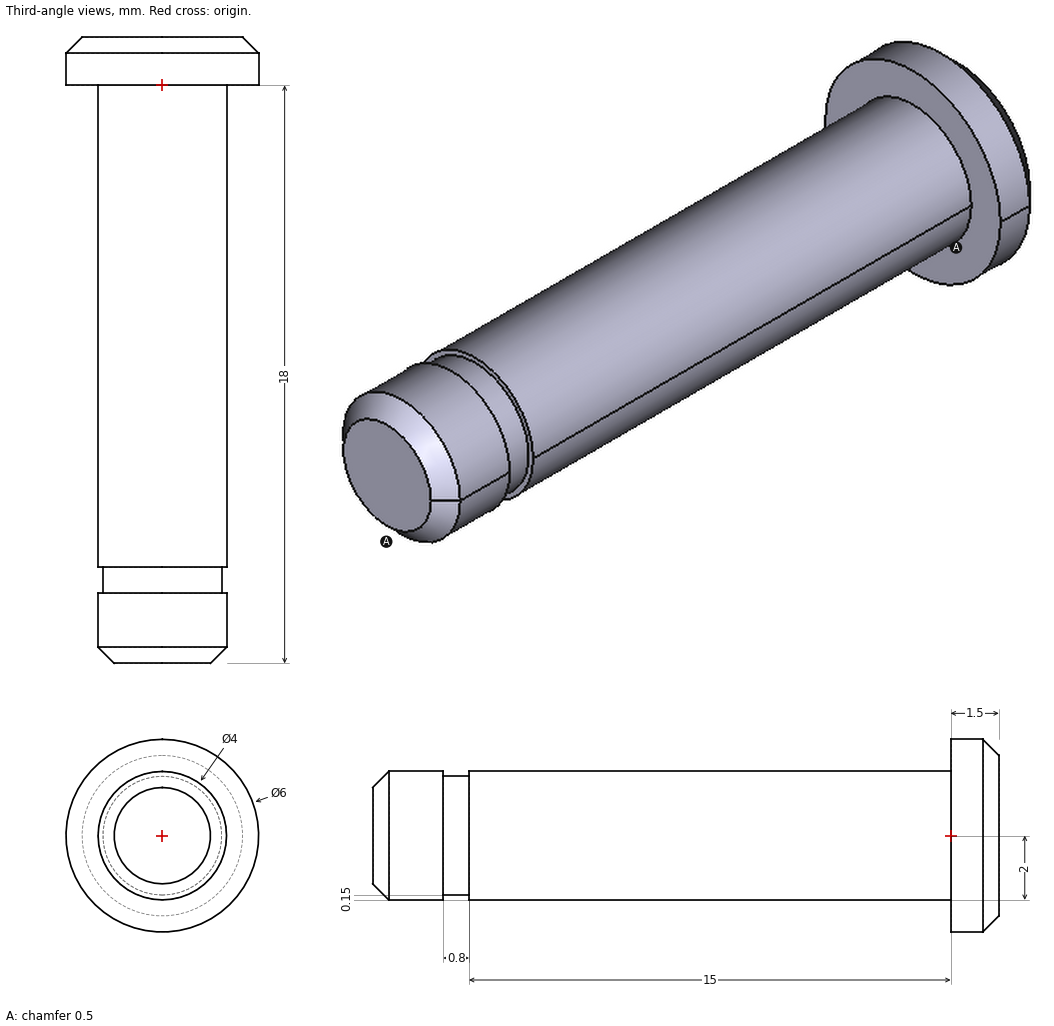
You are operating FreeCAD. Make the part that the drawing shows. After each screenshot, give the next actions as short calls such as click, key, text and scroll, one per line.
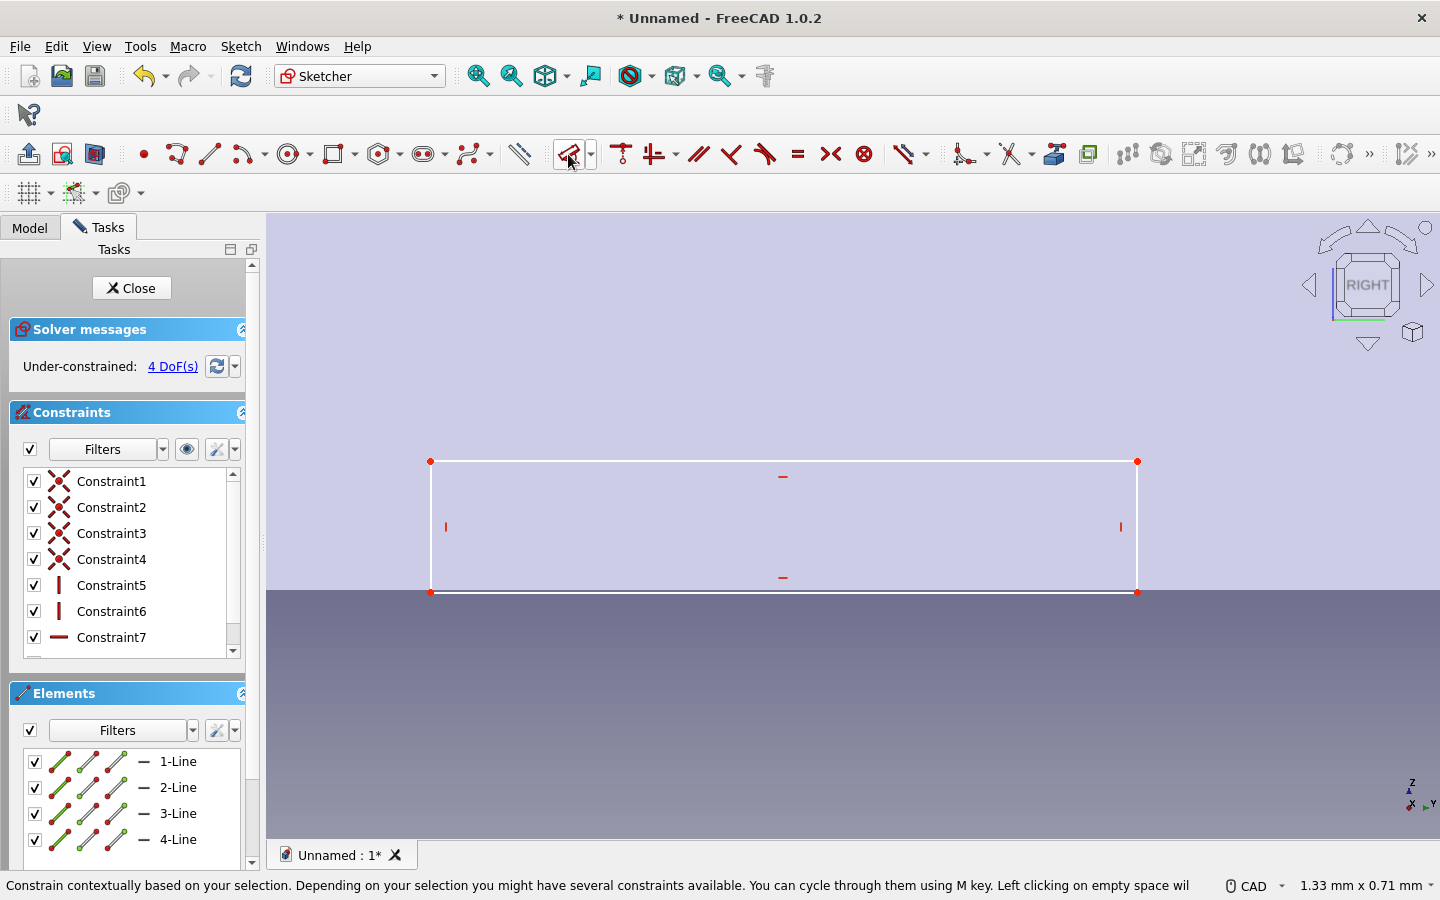
click(431, 593)
click(397, 417)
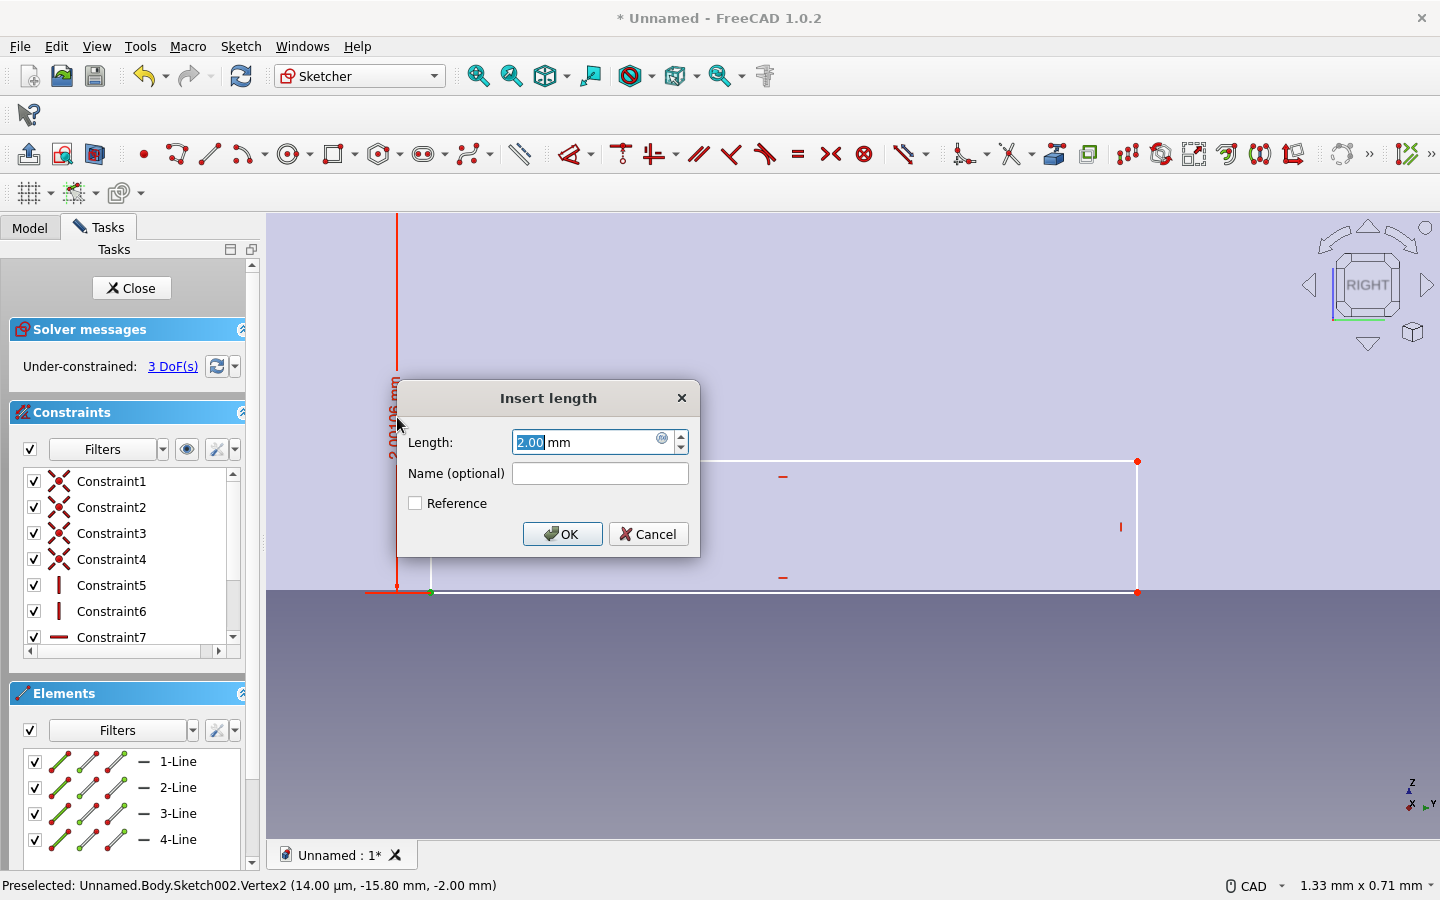
text(2)
key(Return)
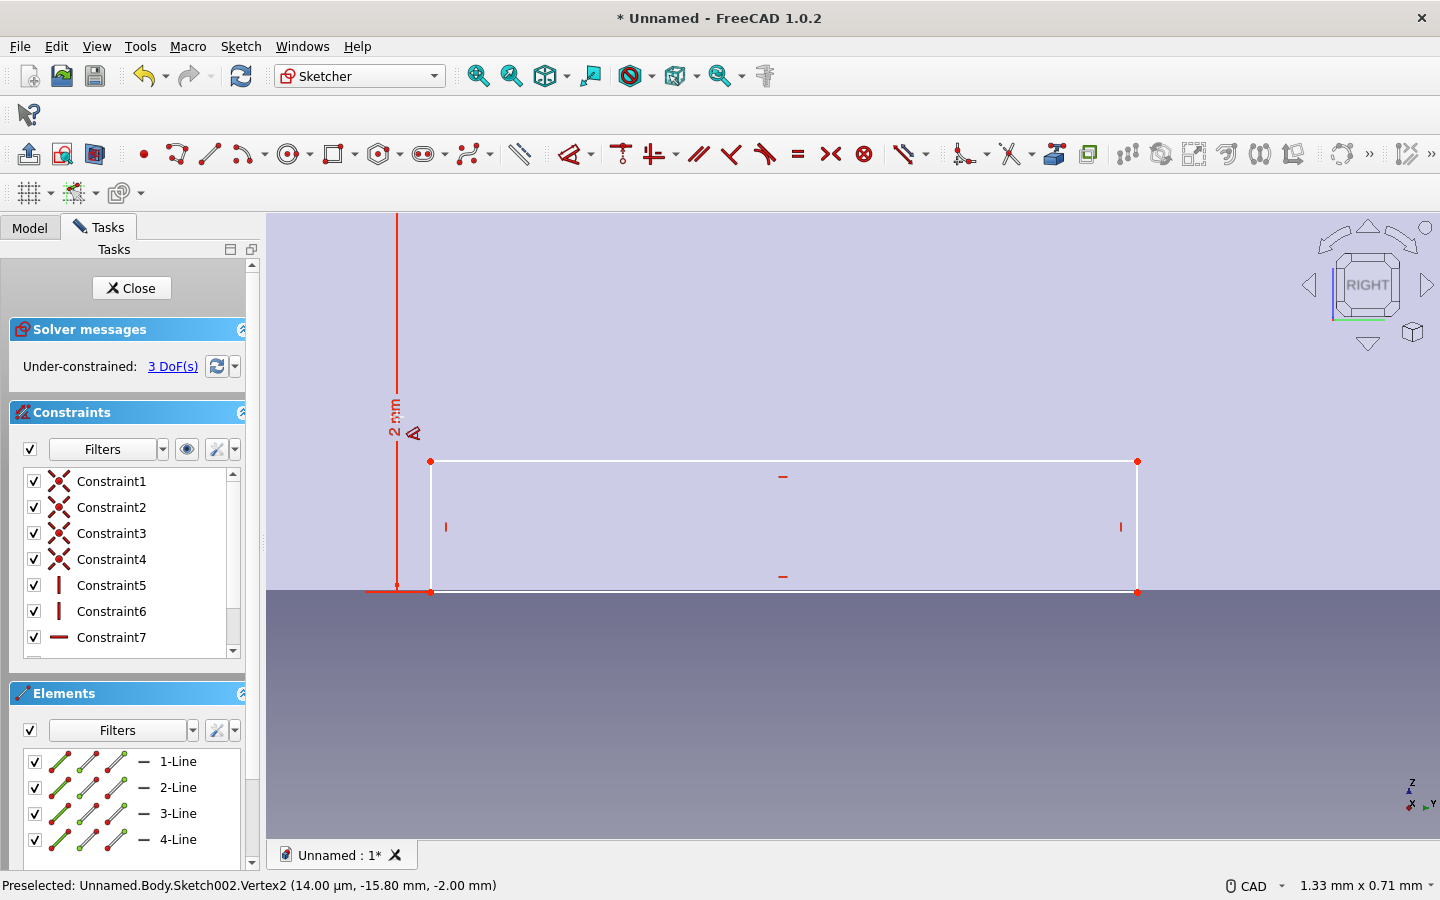
click(643, 592)
click(784, 626)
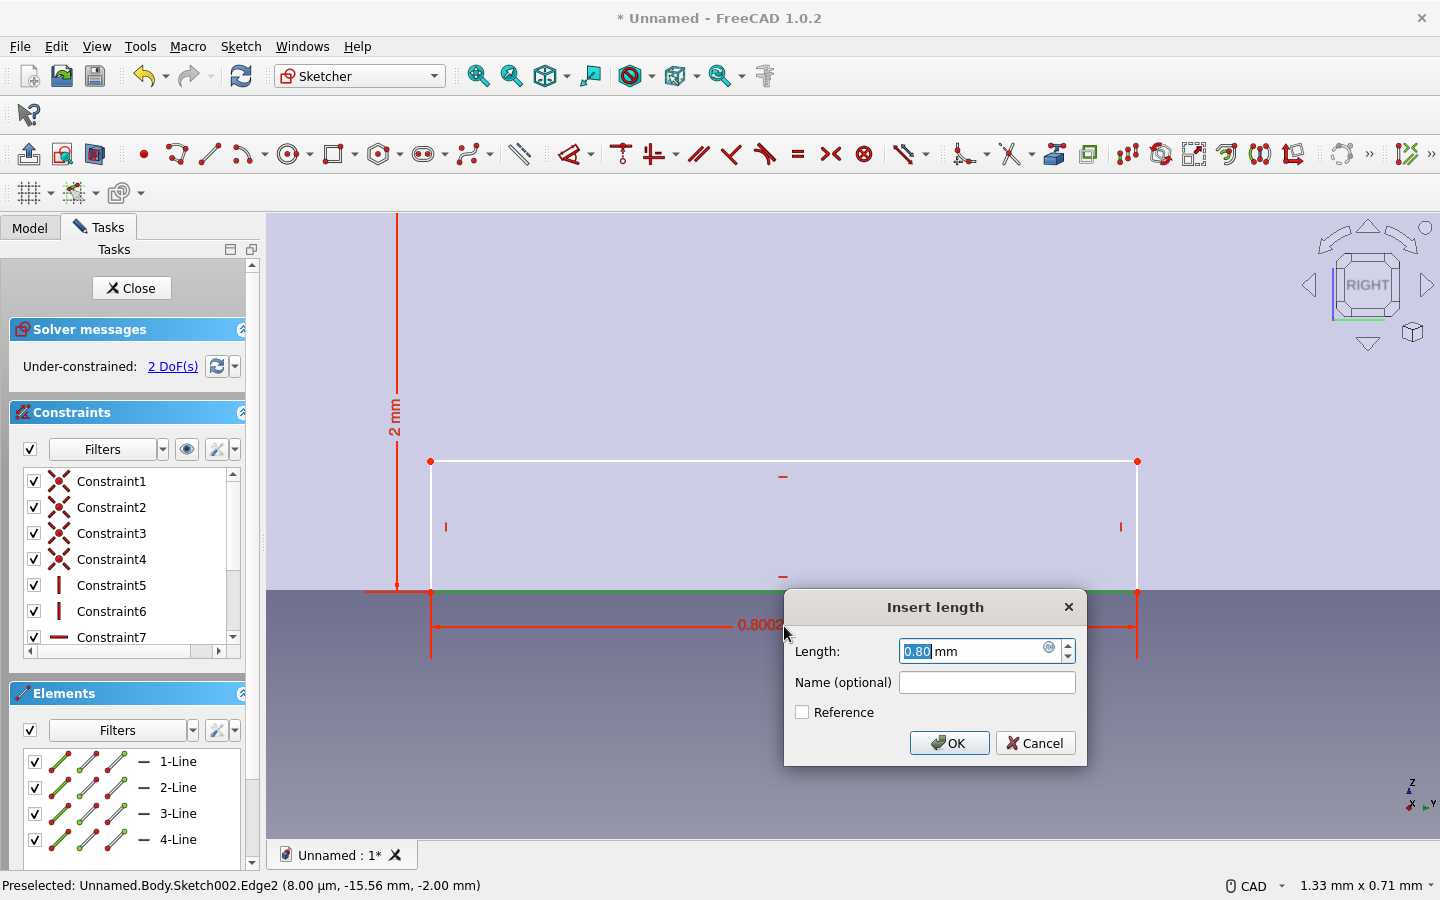
text(0.8)
key(Return)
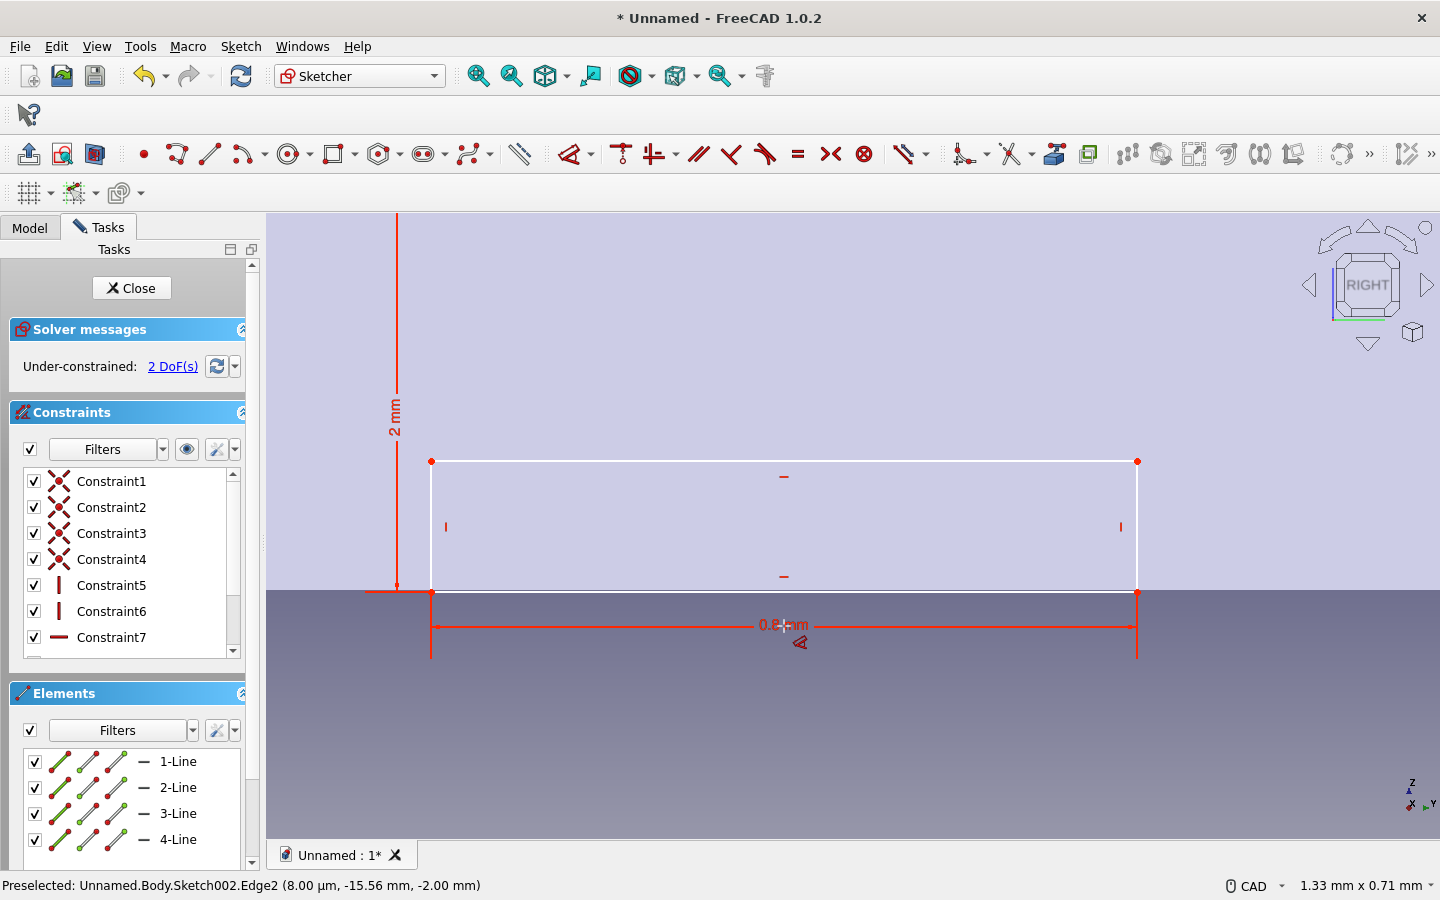
click(1137, 592)
click(1206, 626)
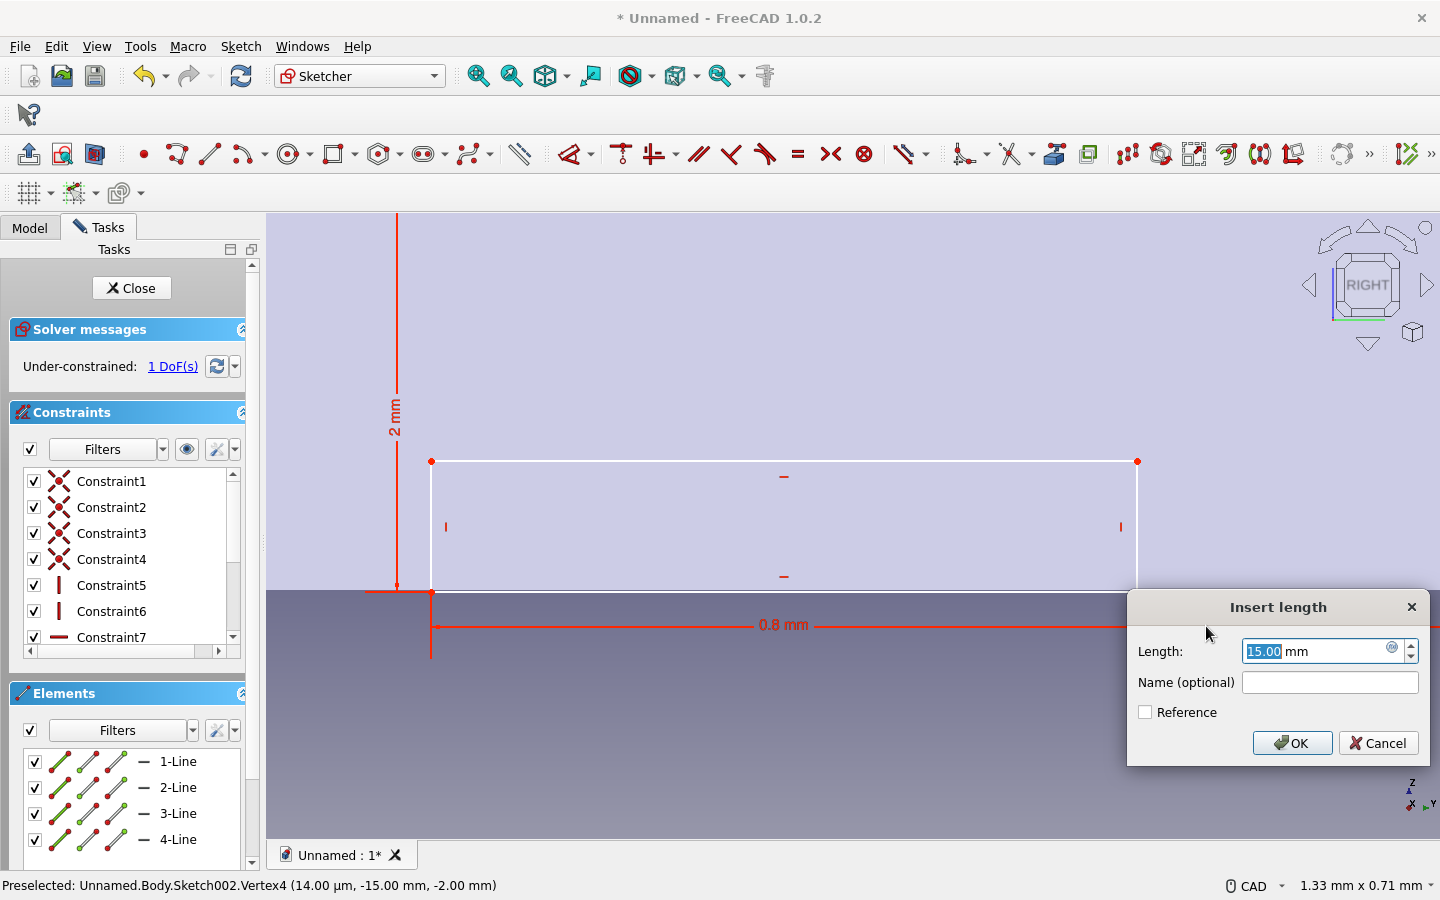
text(15)
key(Return)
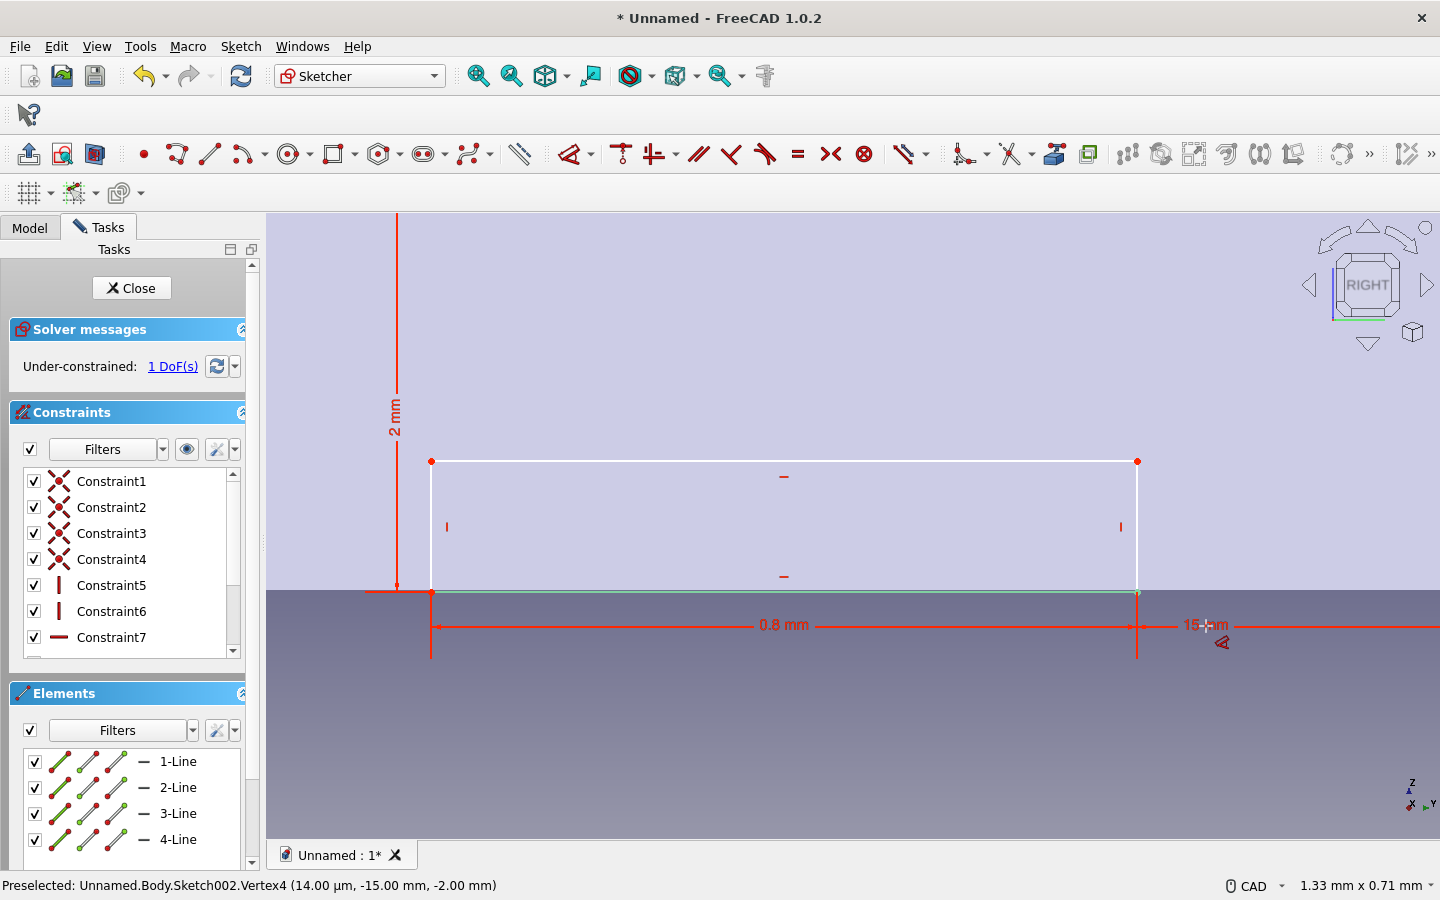
click(431, 500)
click(397, 527)